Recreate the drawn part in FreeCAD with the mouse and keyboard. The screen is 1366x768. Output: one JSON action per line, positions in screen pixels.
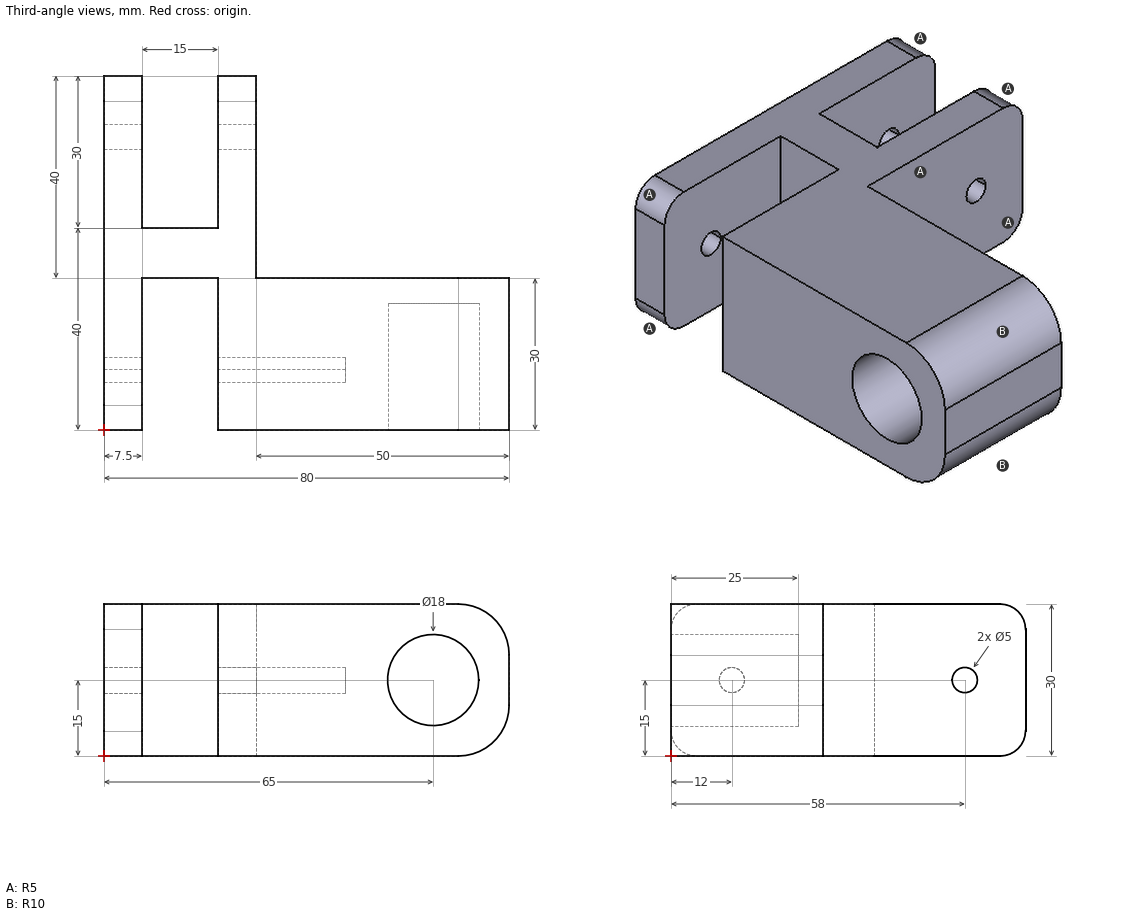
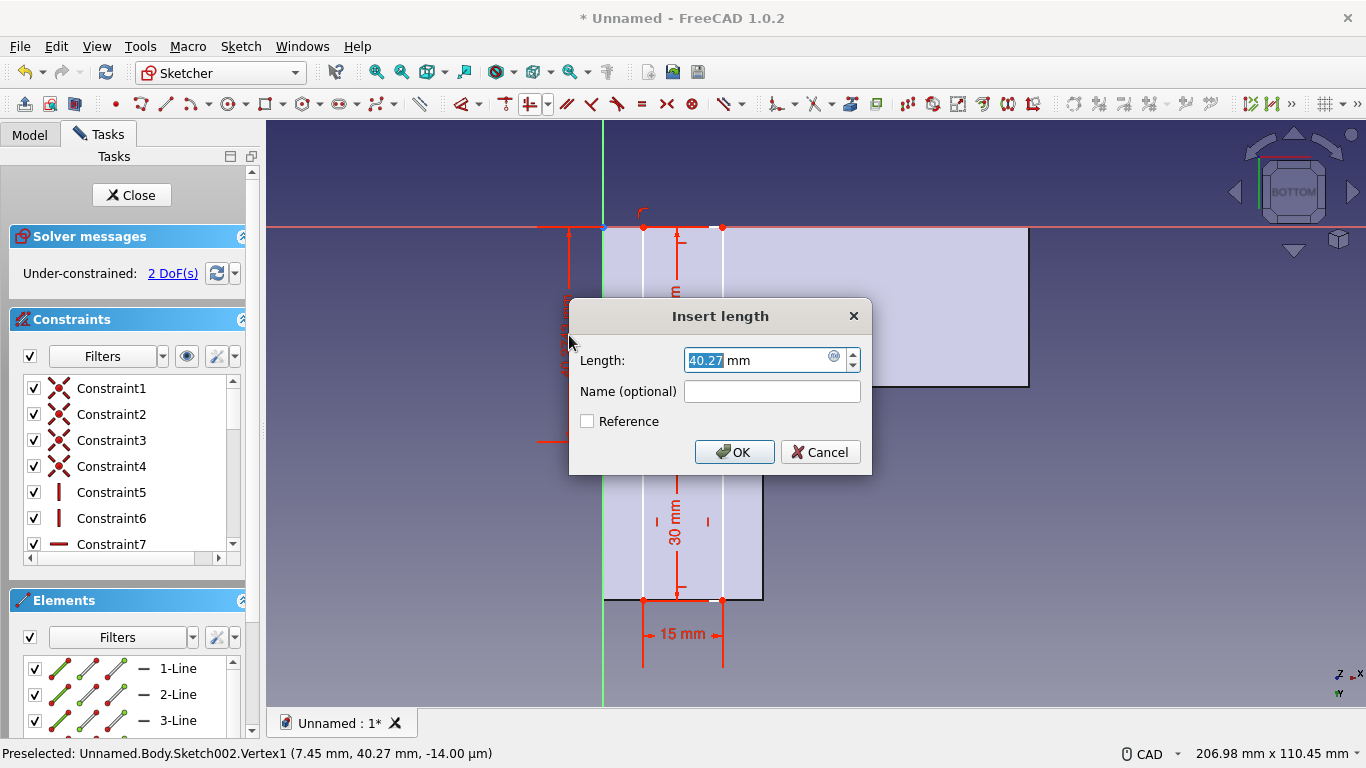
{"action": "type", "text": "40"}
{"action": "key", "text": "Return"}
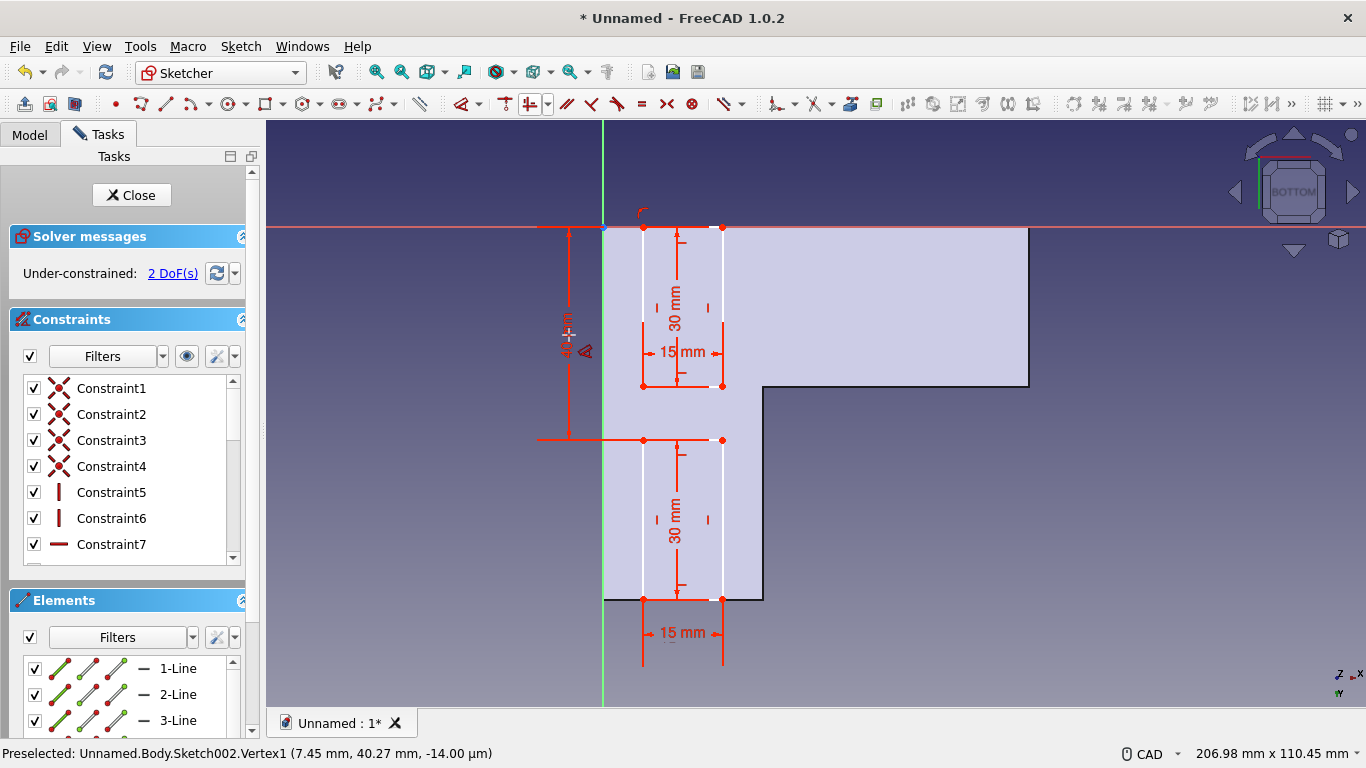
{"action": "left_click", "coordinate": [643, 440]}
{"action": "left_click", "coordinate": [623, 193]}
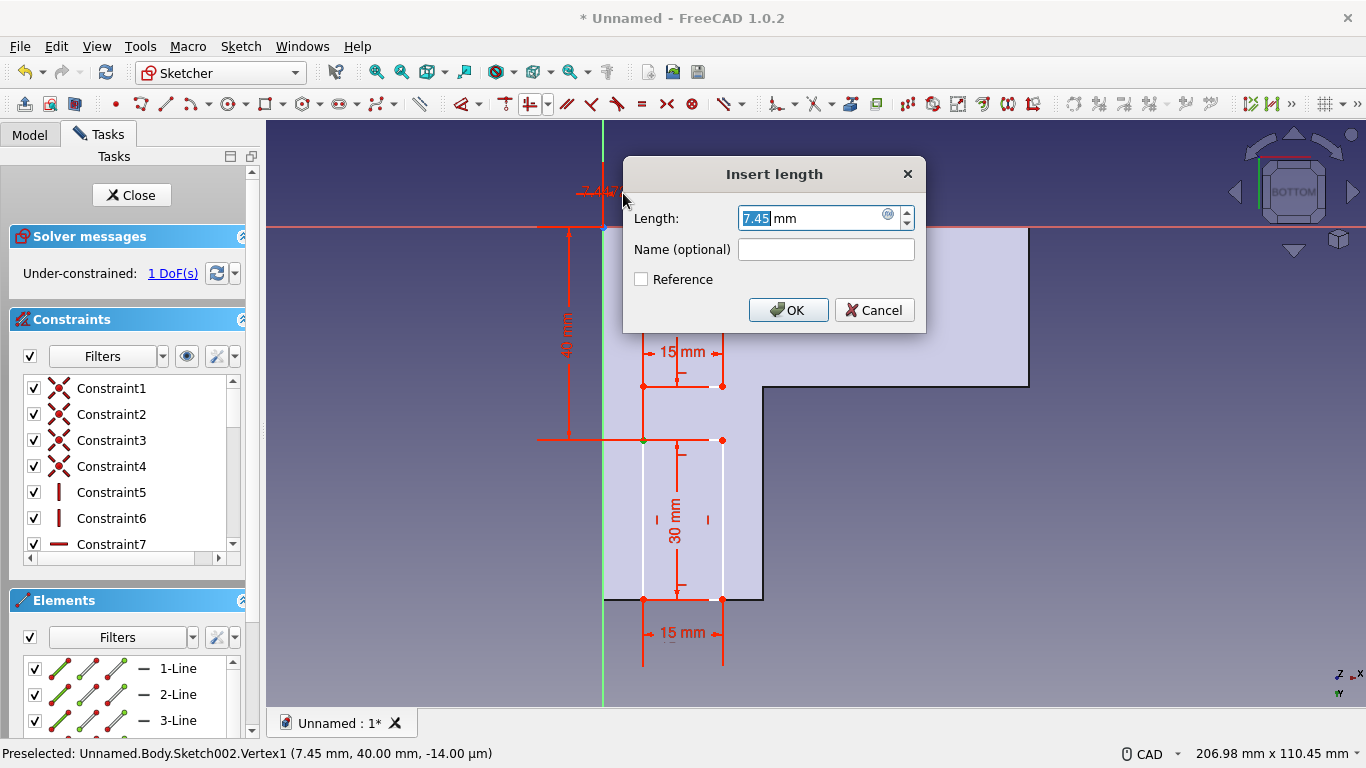
{"action": "type", "text": "7.5"}
{"action": "key", "text": "Return"}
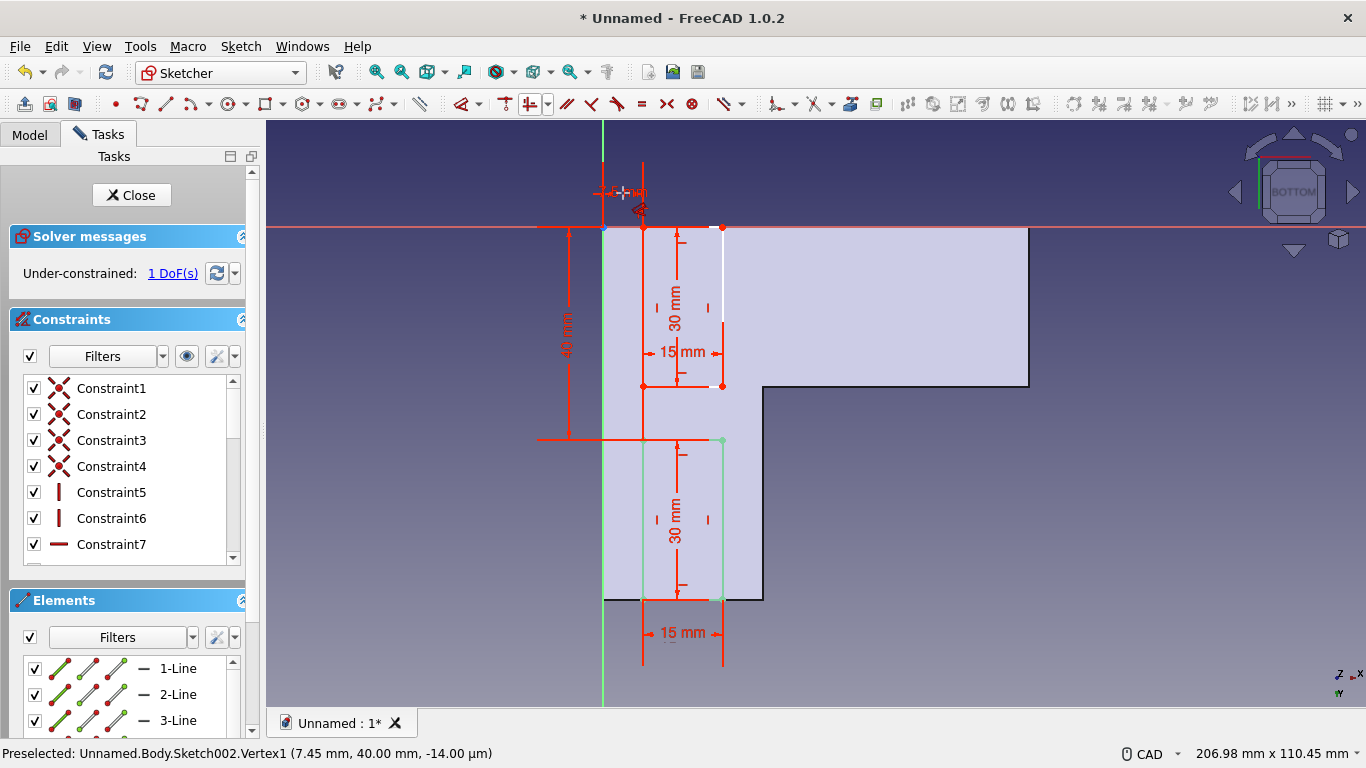
{"action": "left_click", "coordinate": [643, 227]}
{"action": "left_click", "coordinate": [623, 261]}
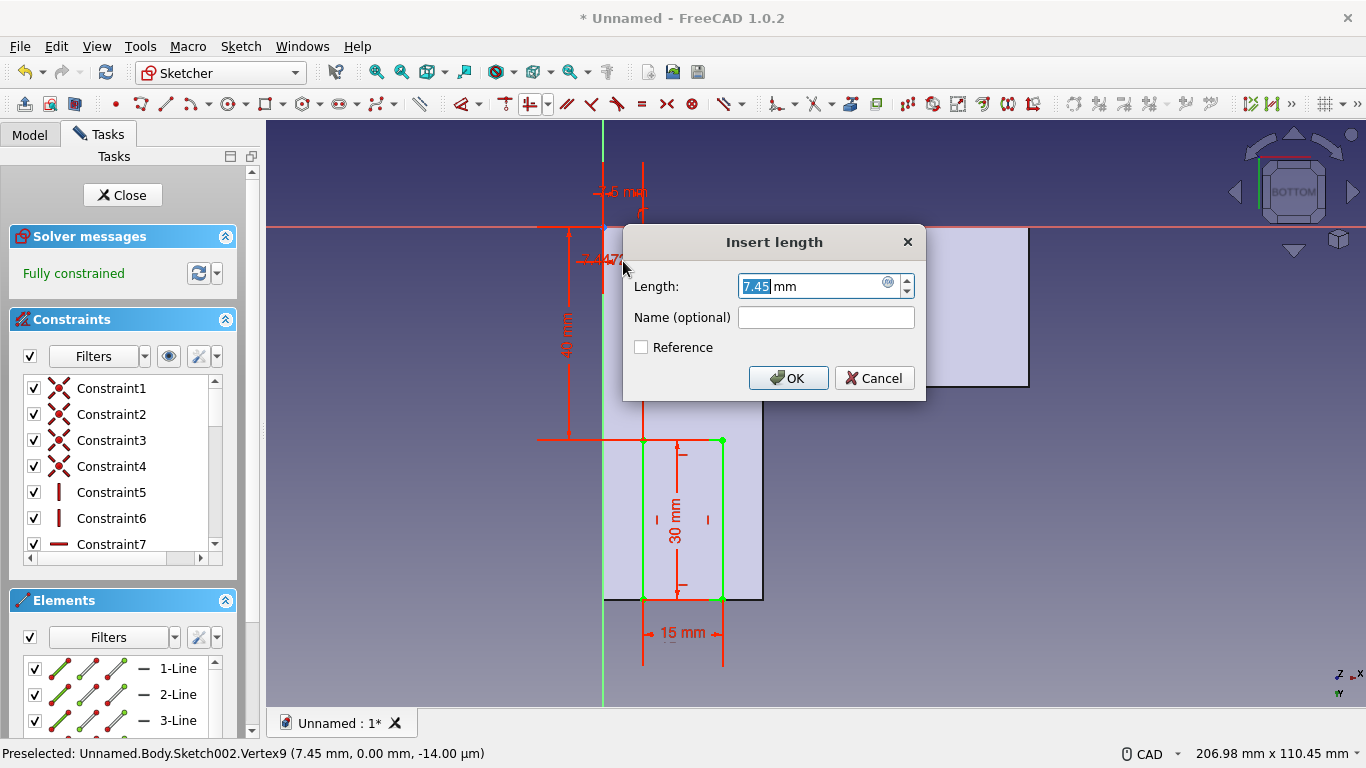
{"action": "type", "text": "7.5"}
{"action": "key", "text": "Return"}
{"action": "key", "text": "Escape"}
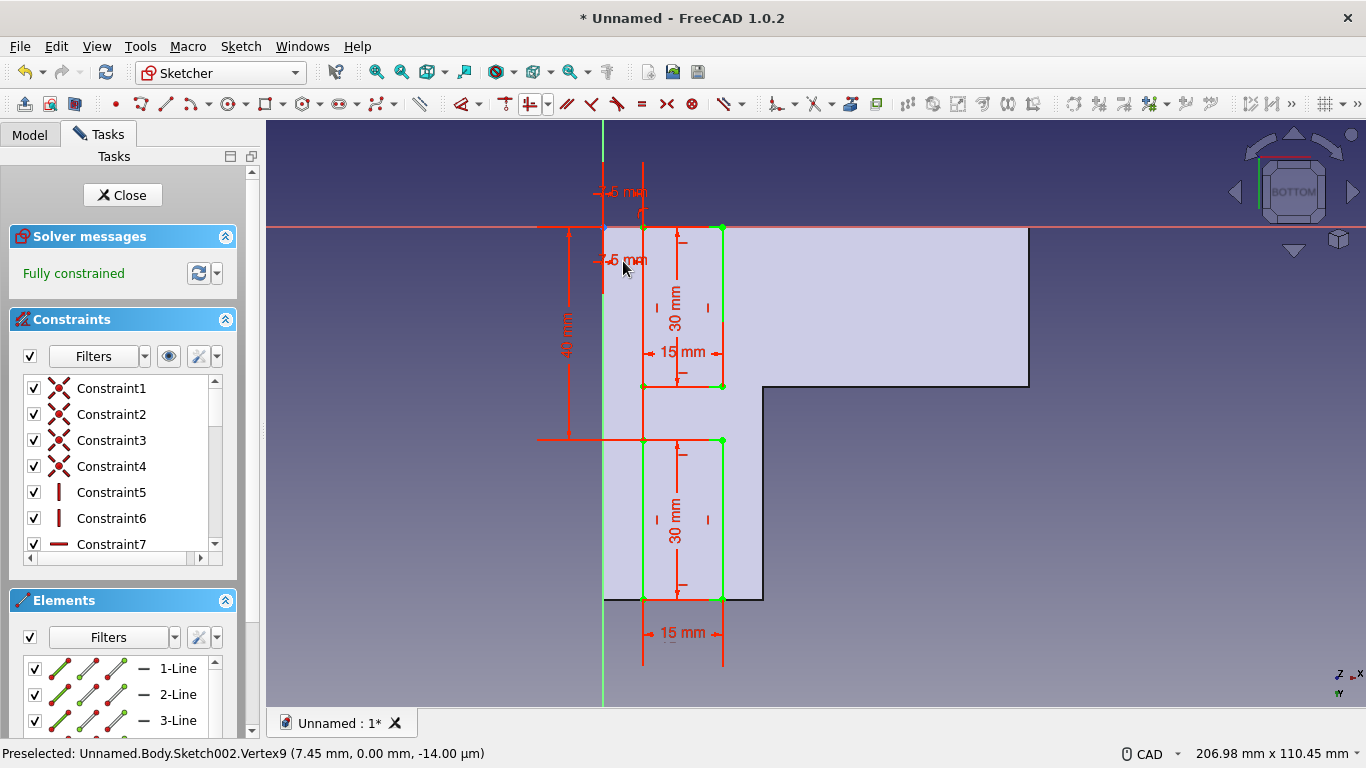
{"action": "left_click", "coordinate": [123, 195]}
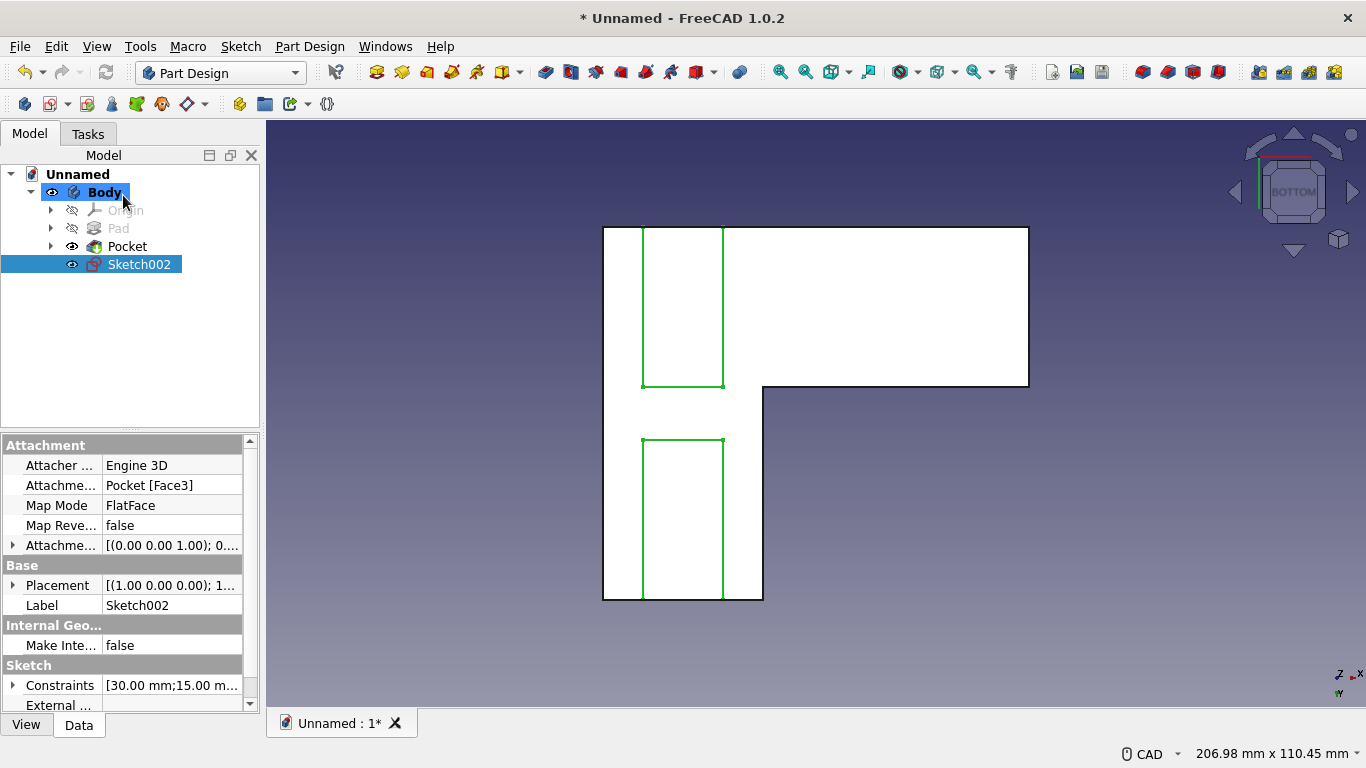
{"action": "left_click", "coordinate": [546, 72]}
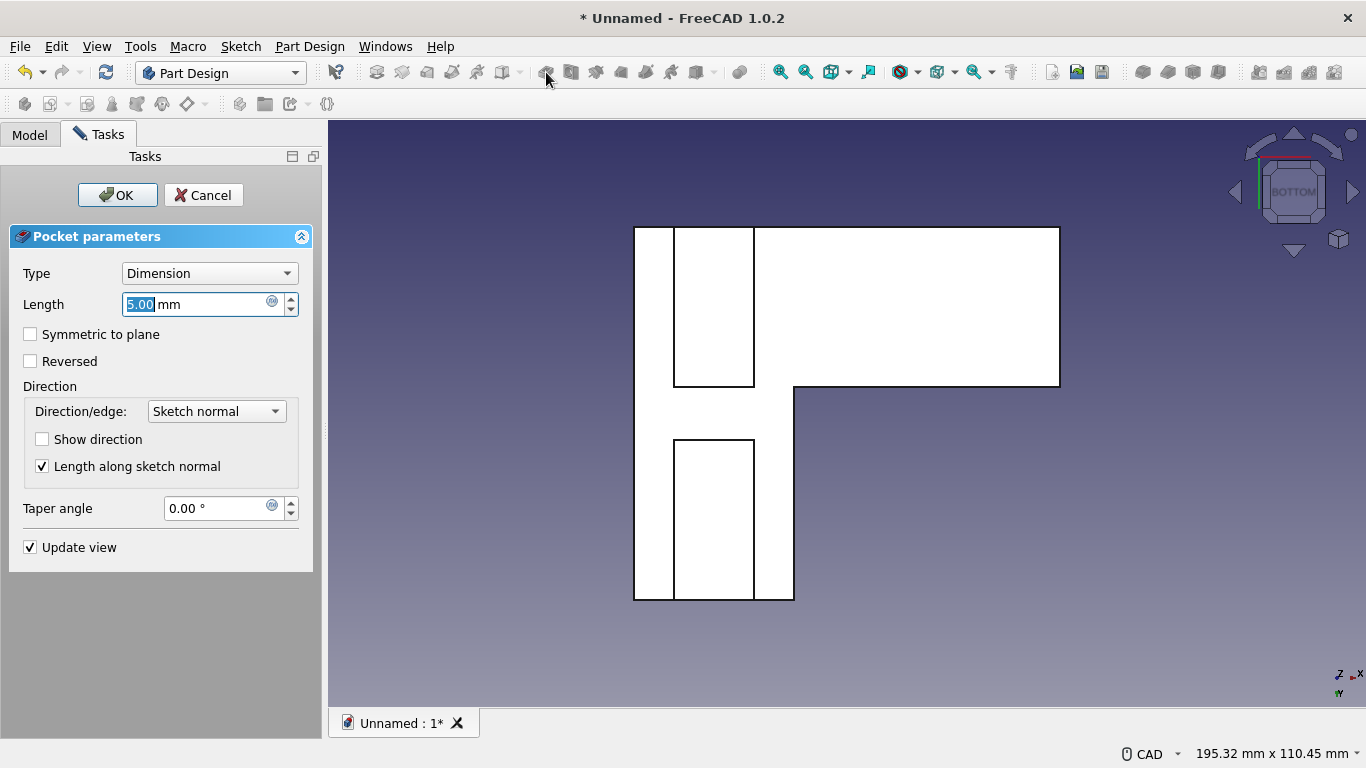
{"action": "left_click", "coordinate": [210, 274]}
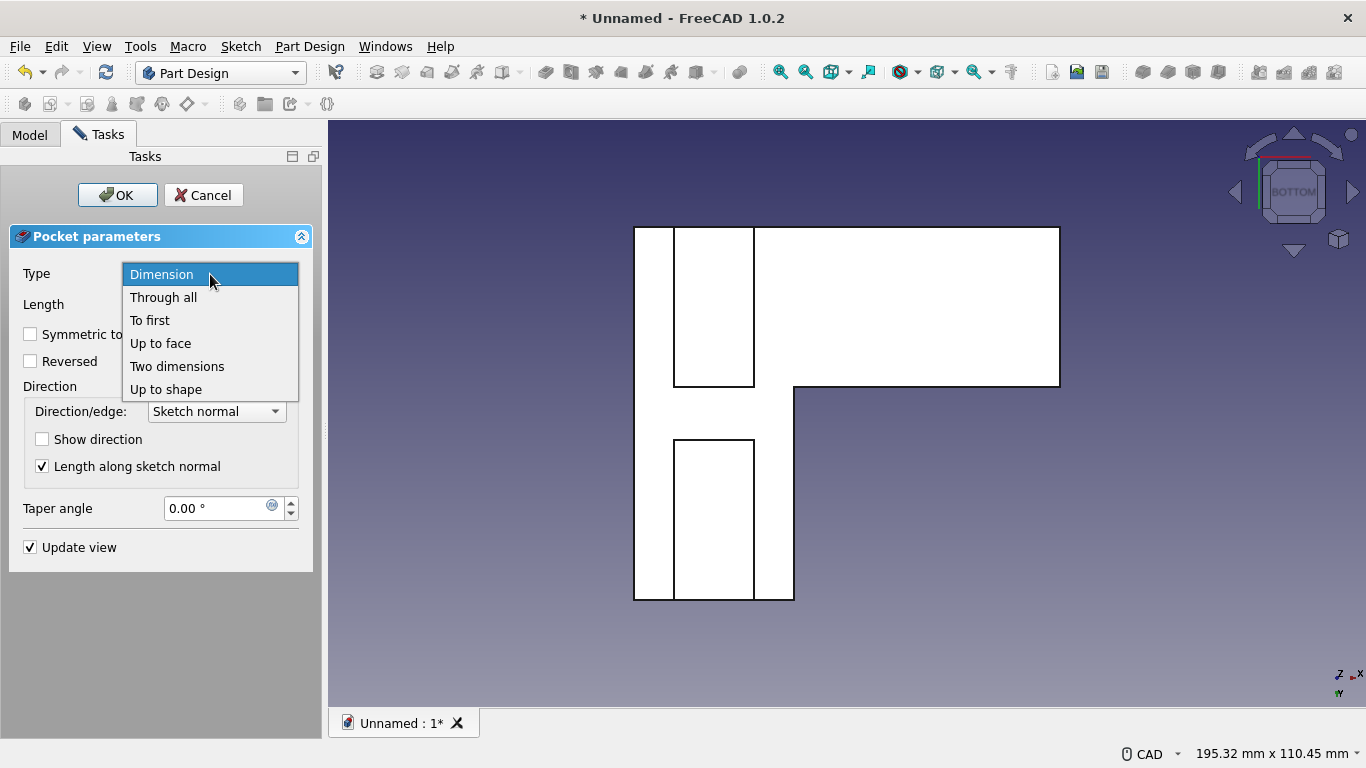
{"action": "left_click", "coordinate": [208, 298]}